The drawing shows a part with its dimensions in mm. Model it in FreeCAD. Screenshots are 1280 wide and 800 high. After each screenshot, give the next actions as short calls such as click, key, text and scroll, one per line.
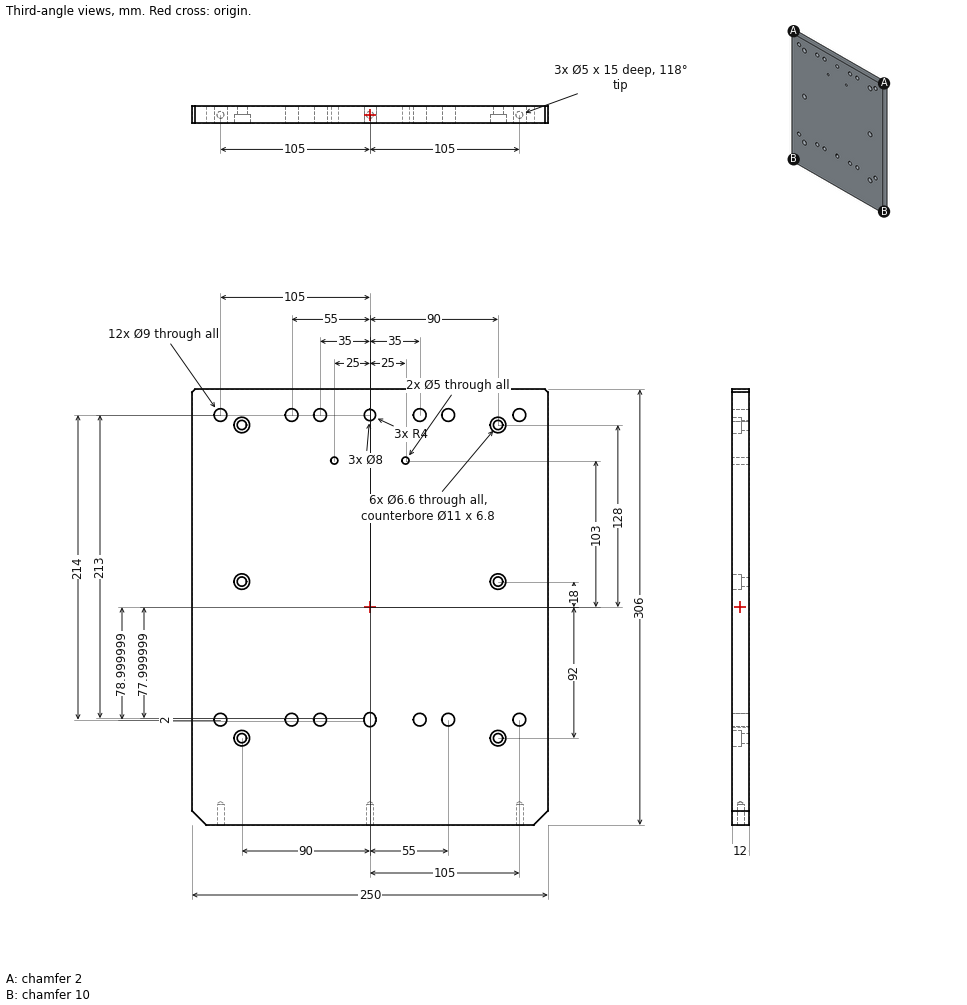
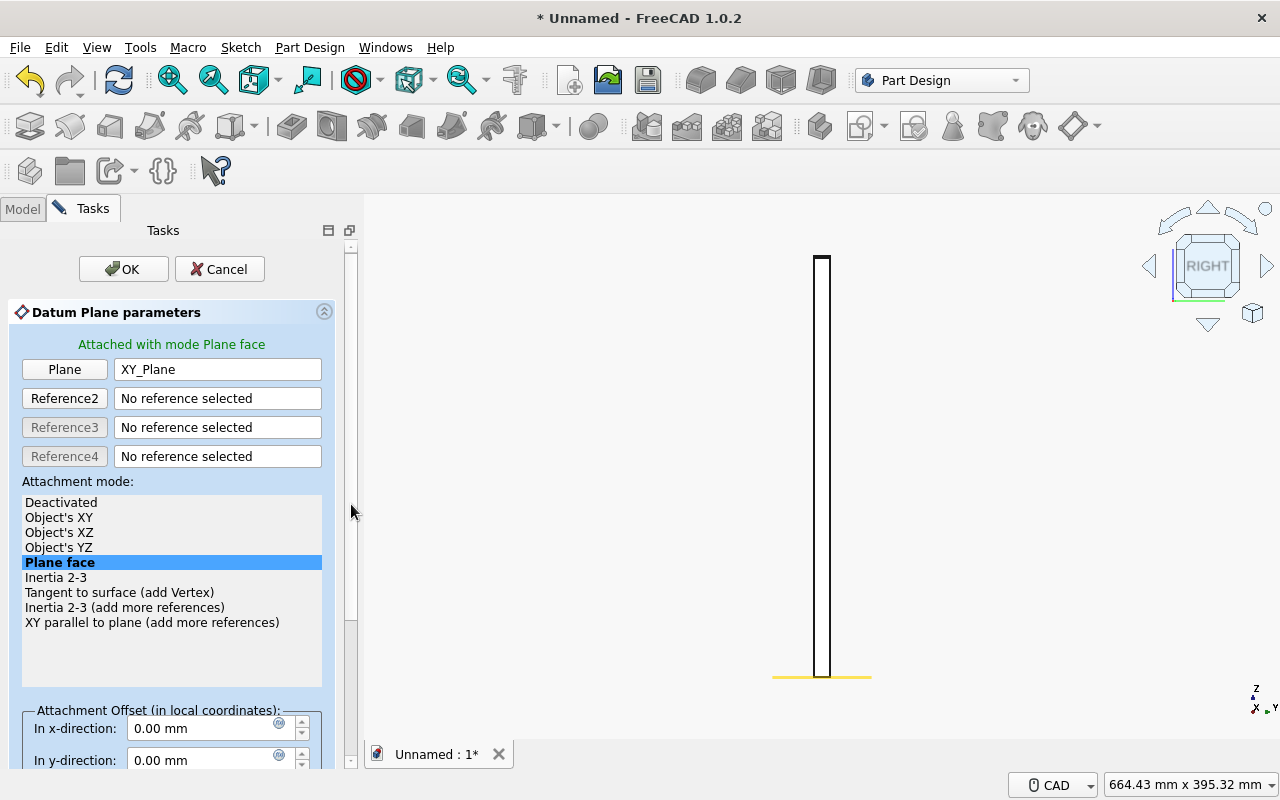
click(124, 269)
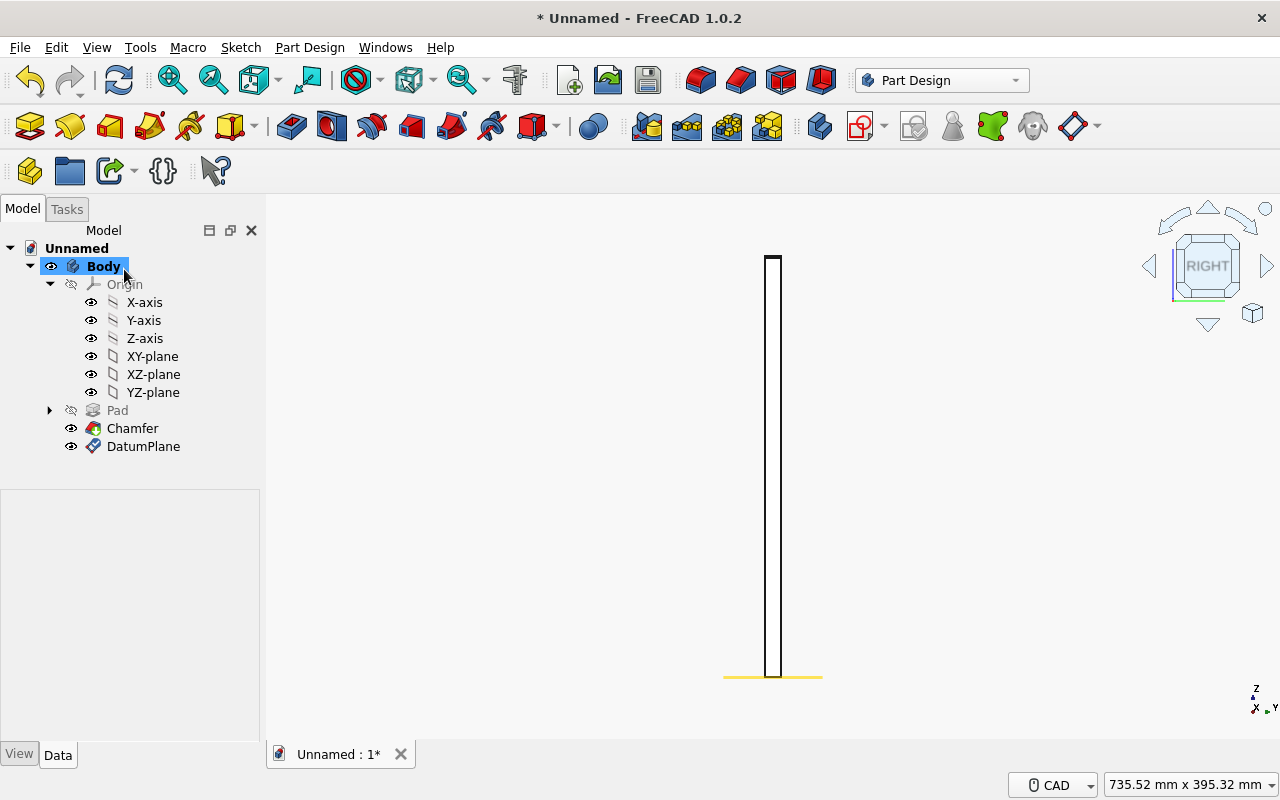
click(116, 446)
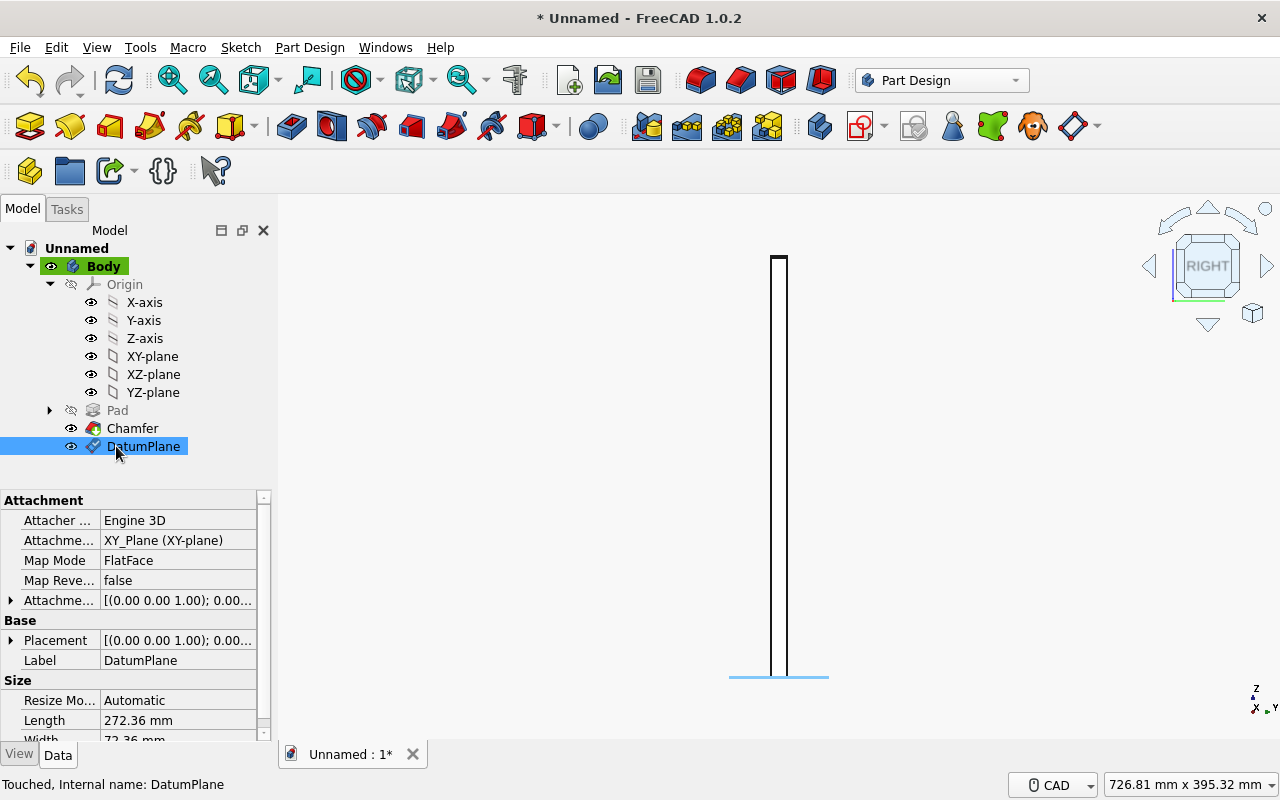
click(860, 126)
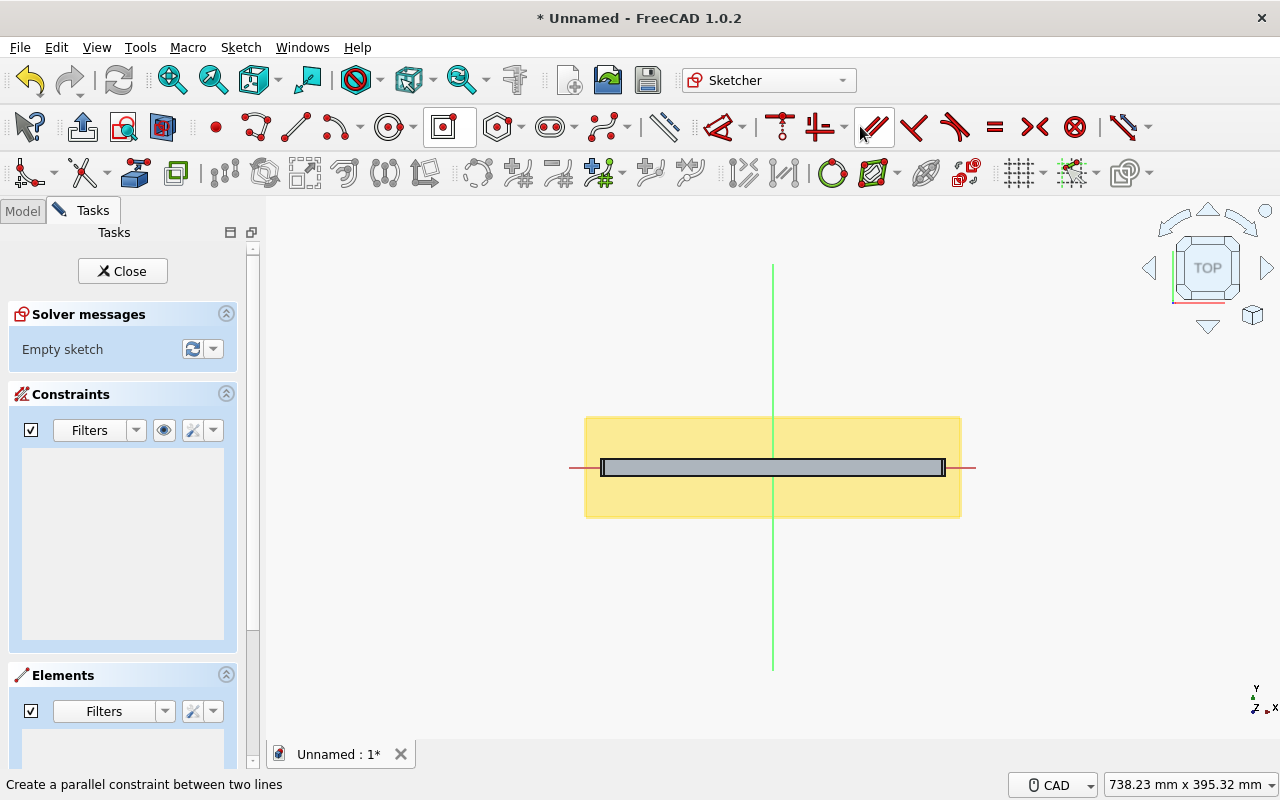
click(164, 128)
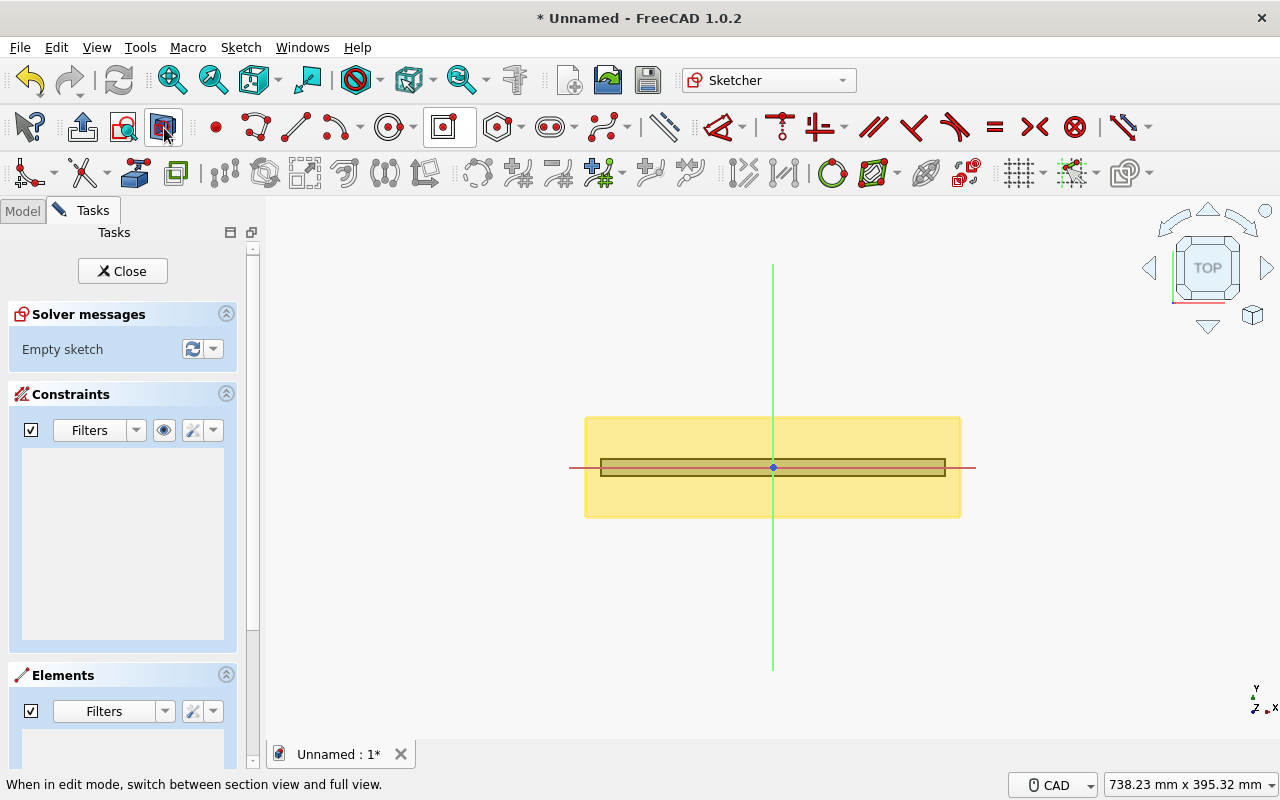
scroll(856, 467, up, 3)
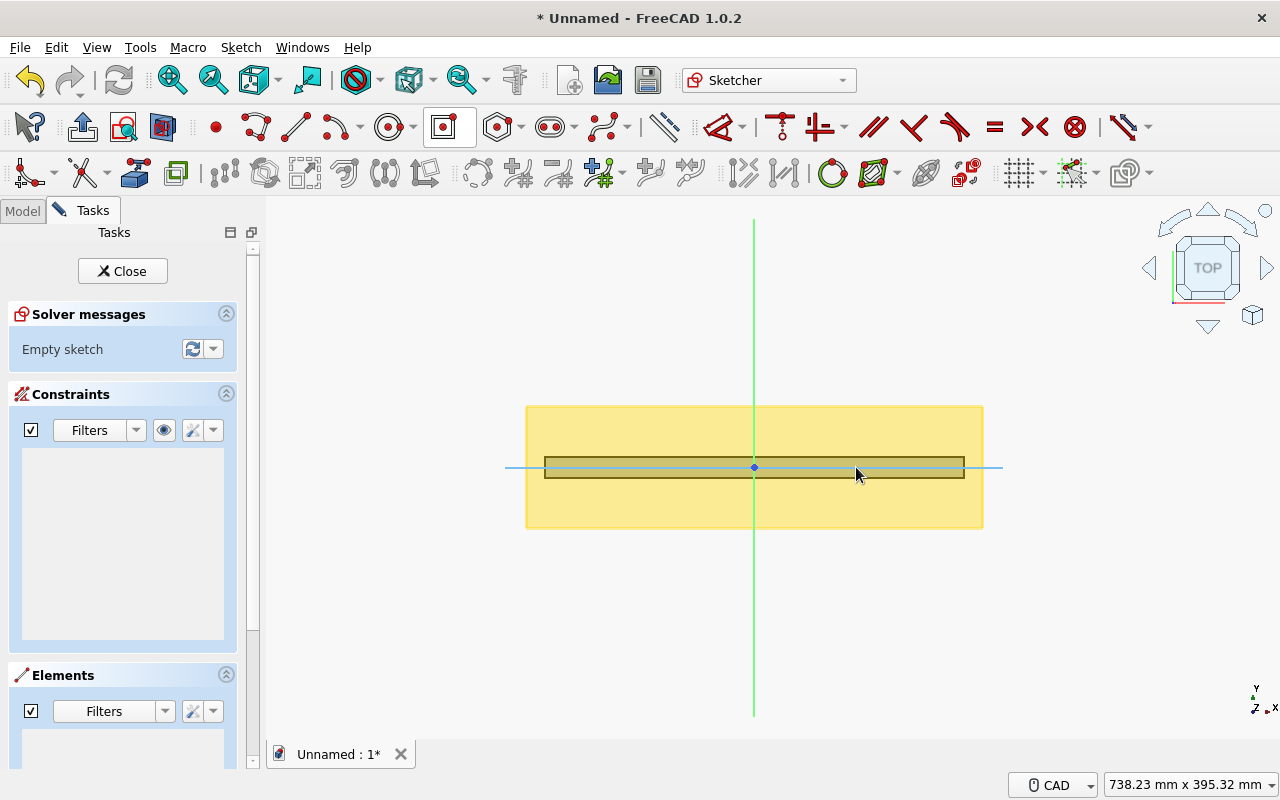
click(390, 128)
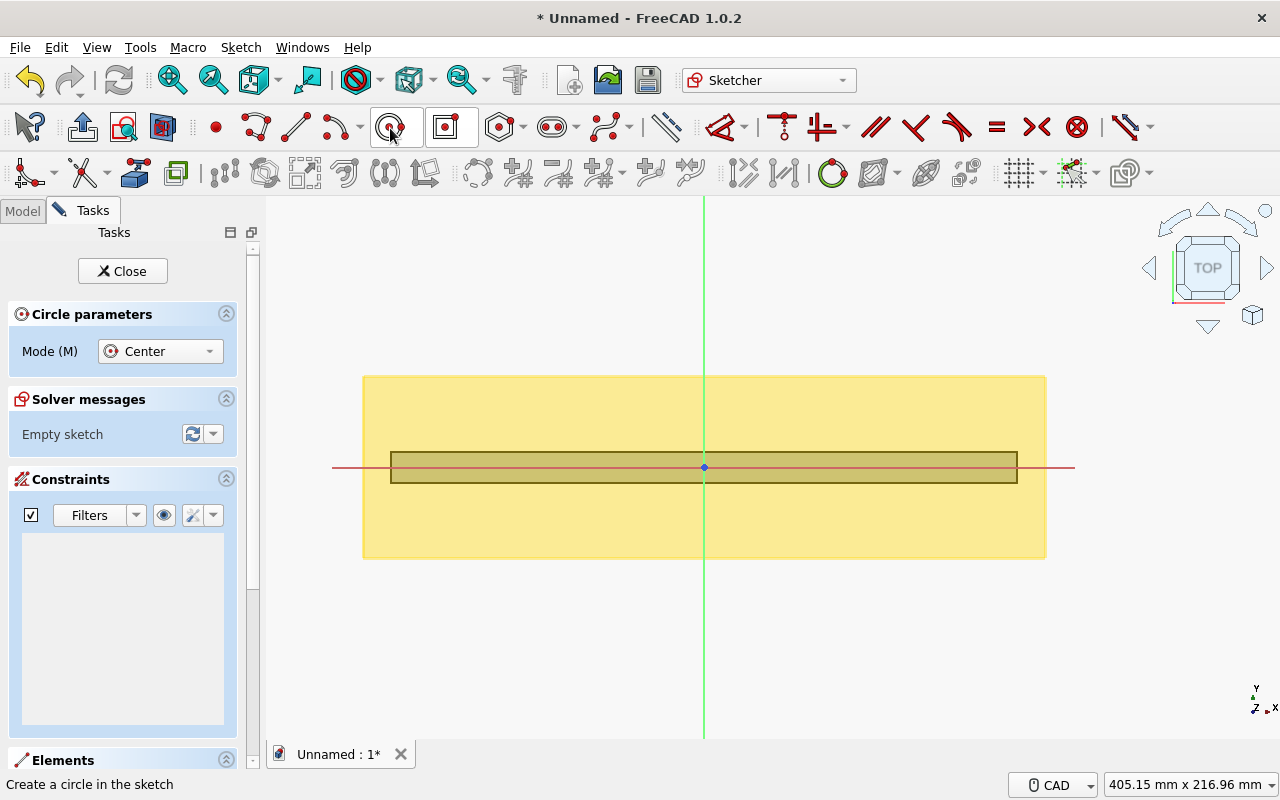
scroll(967, 467, up, 7)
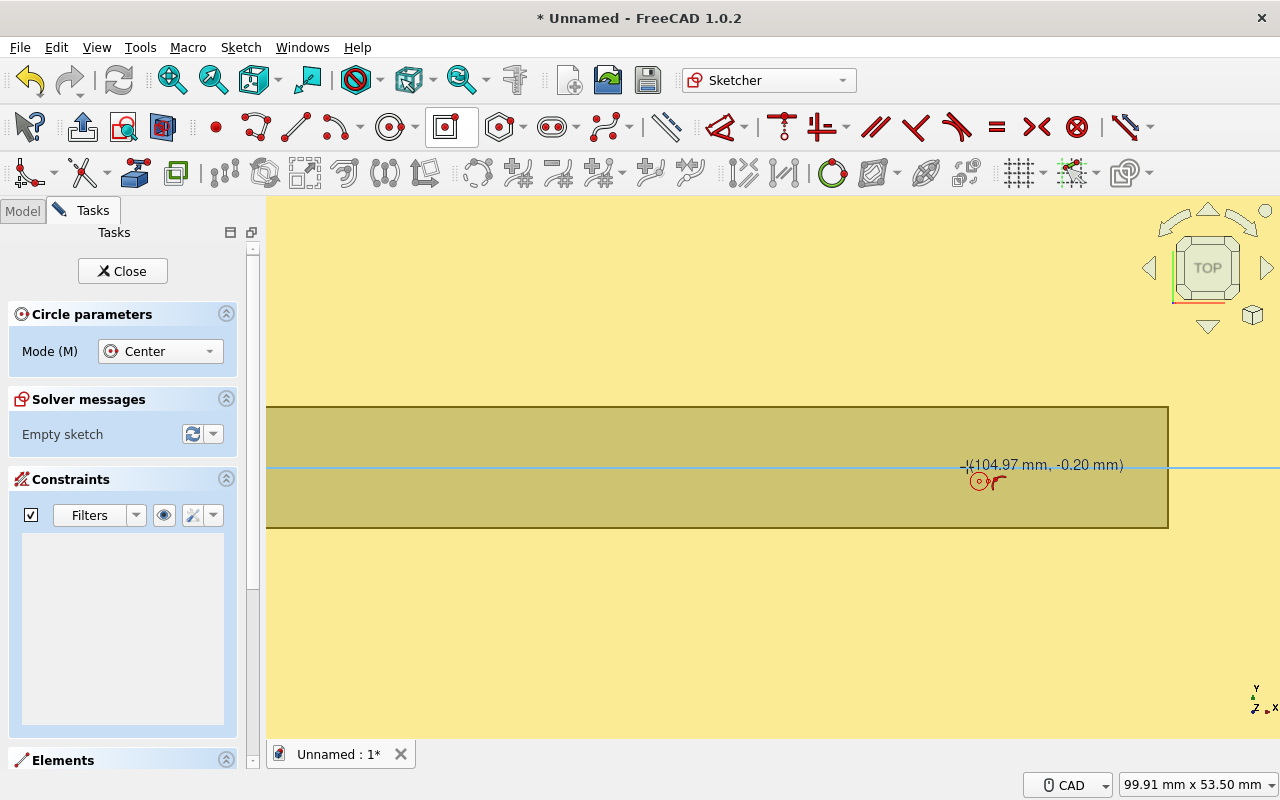
scroll(968, 468, down, 7)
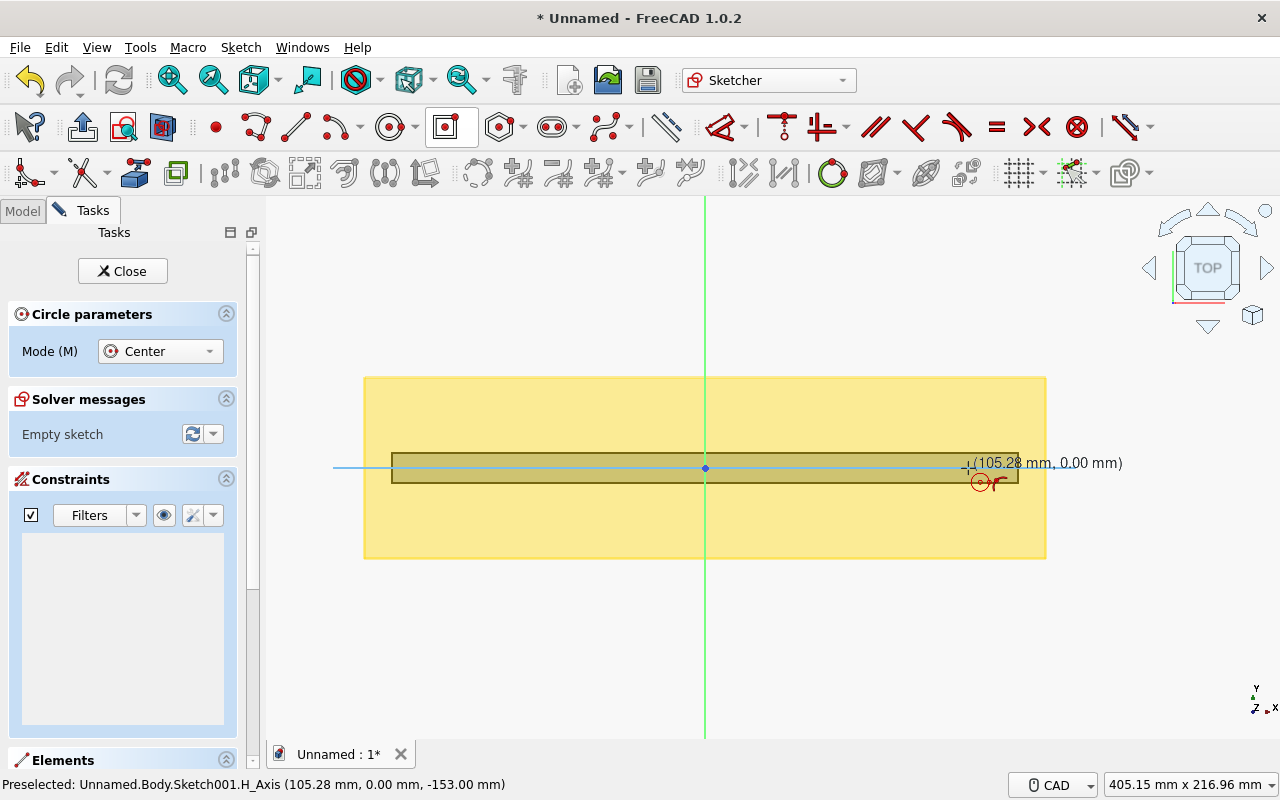
click(968, 468)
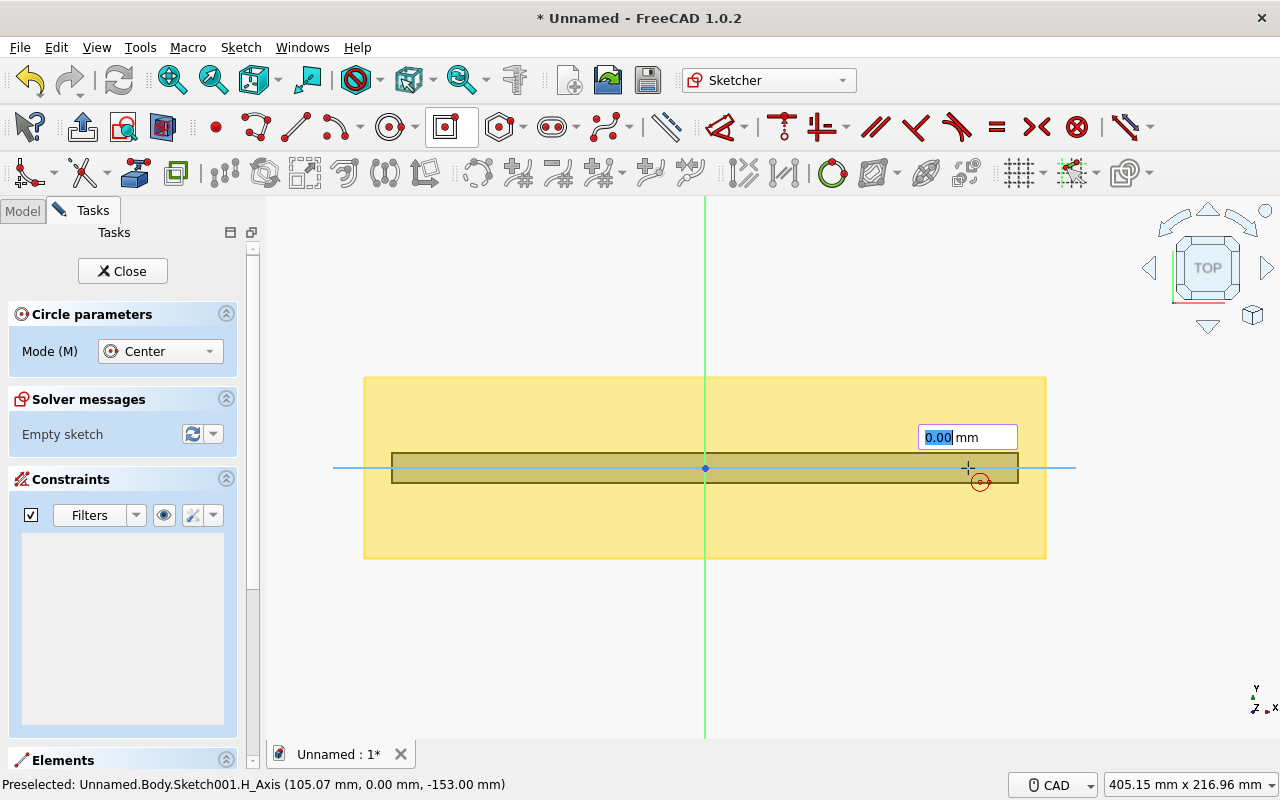
scroll(966, 474, up, 5)
move(964, 473)